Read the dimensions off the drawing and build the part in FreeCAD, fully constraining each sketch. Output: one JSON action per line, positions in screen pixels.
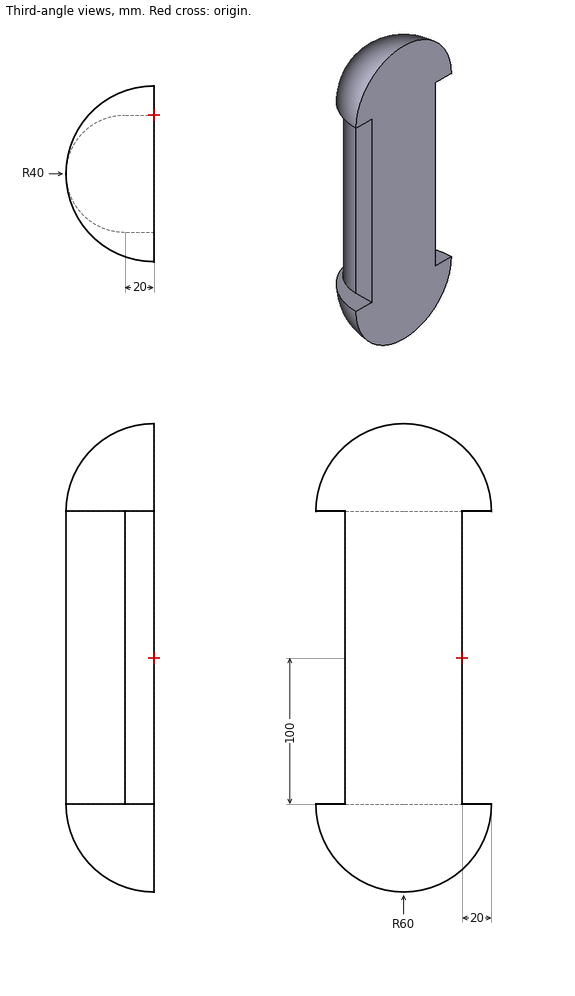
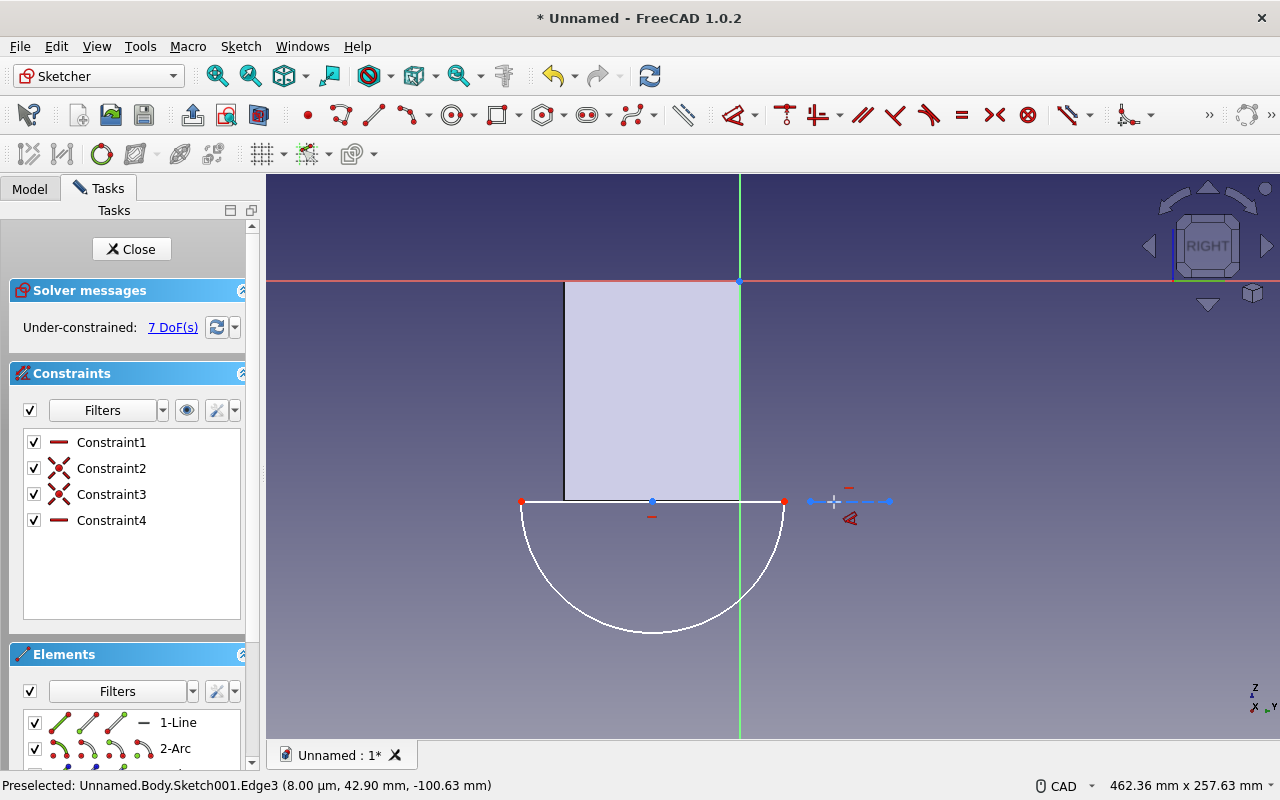
{"action": "left_click", "coordinate": [575, 608]}
{"action": "left_click", "coordinate": [556, 634]}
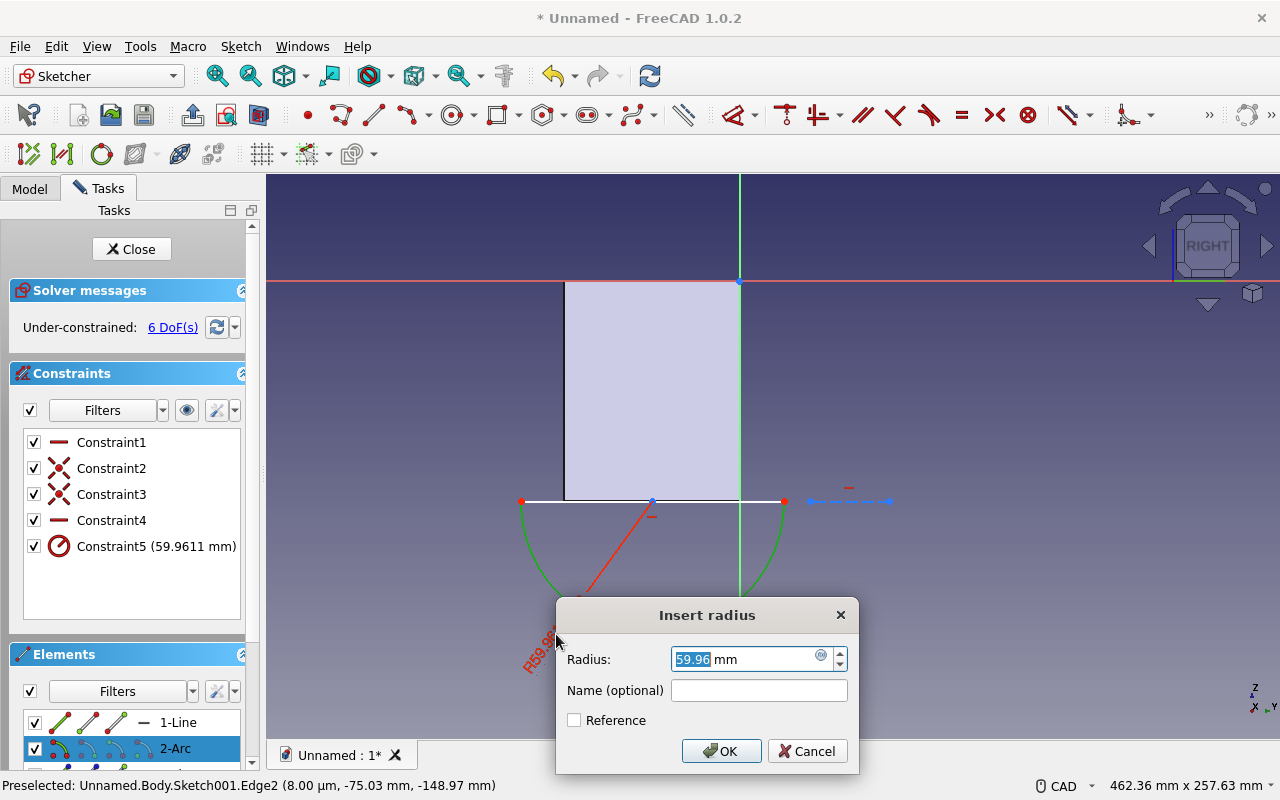
{"action": "type", "text": "60"}
{"action": "key", "text": "Return"}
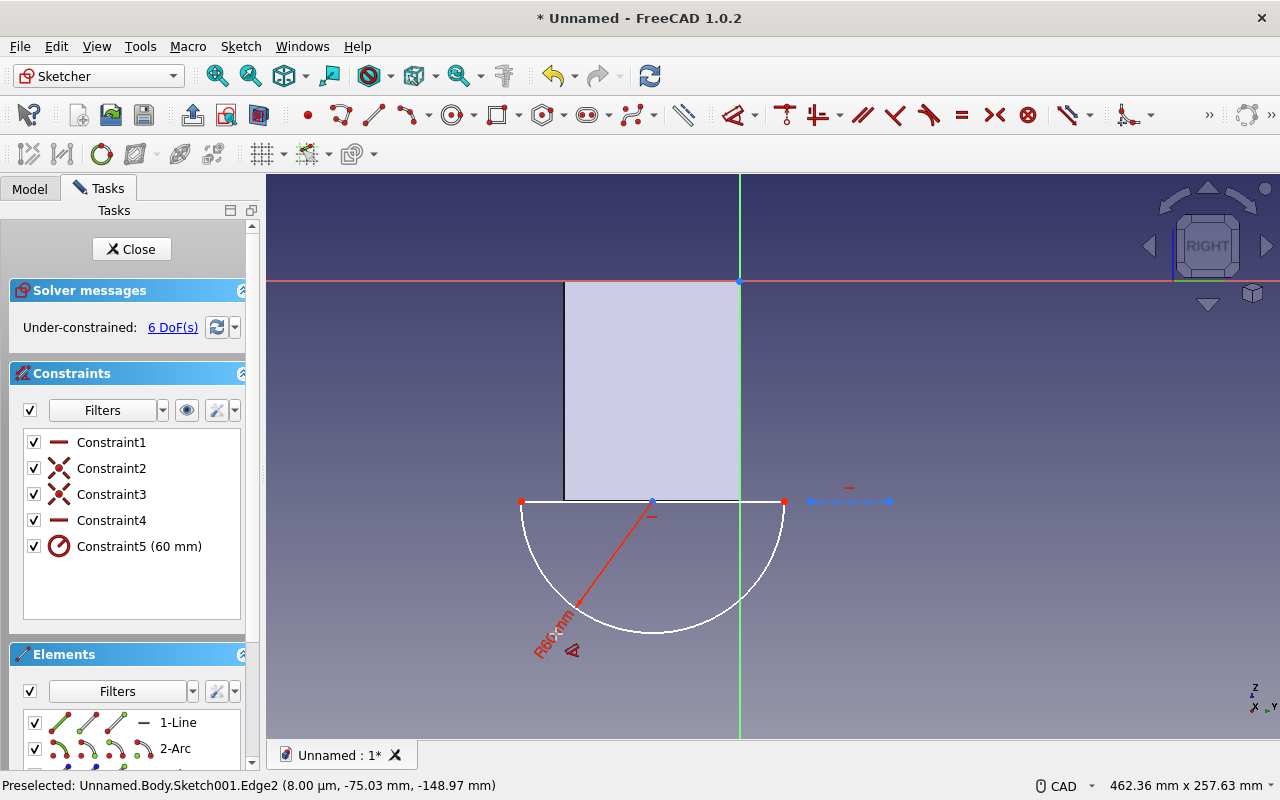
{"action": "left_click", "coordinate": [784, 502]}
{"action": "left_click", "coordinate": [762, 247]}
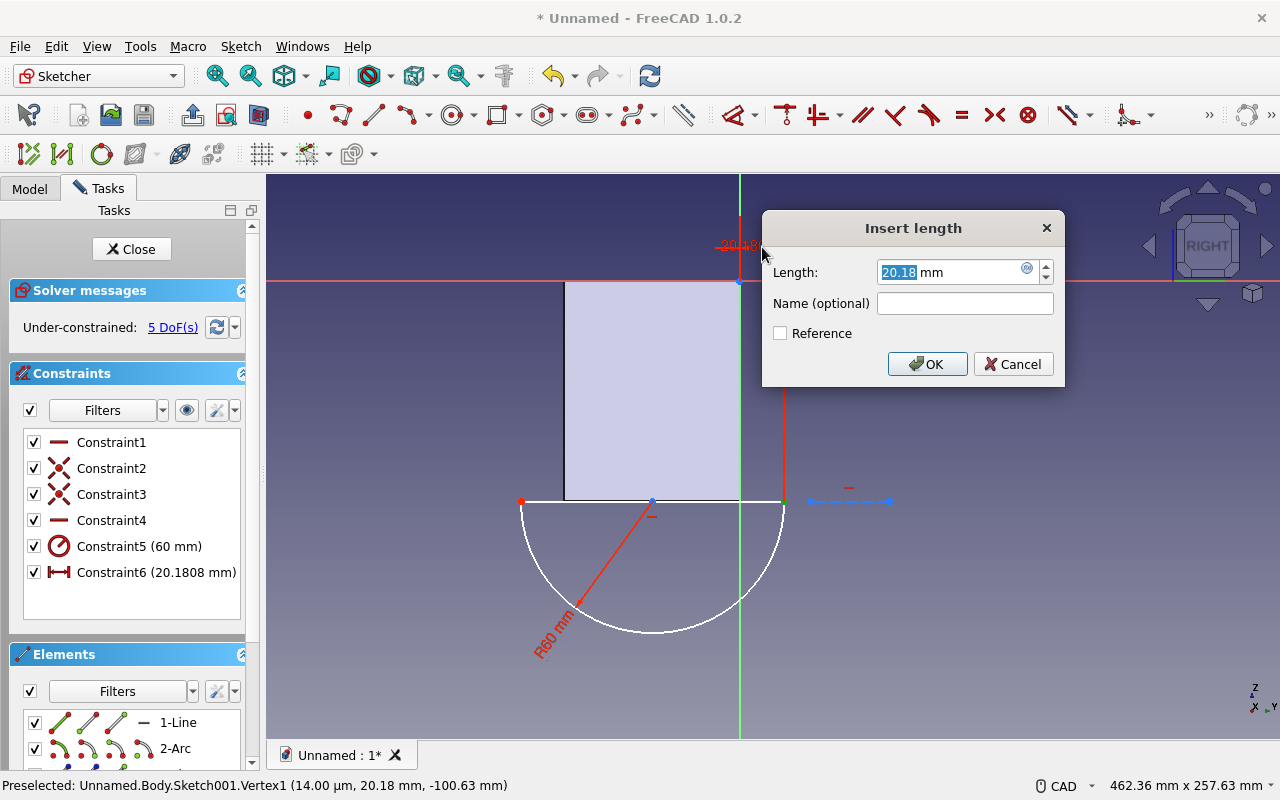
{"action": "type", "text": "20"}
{"action": "key", "text": "Return"}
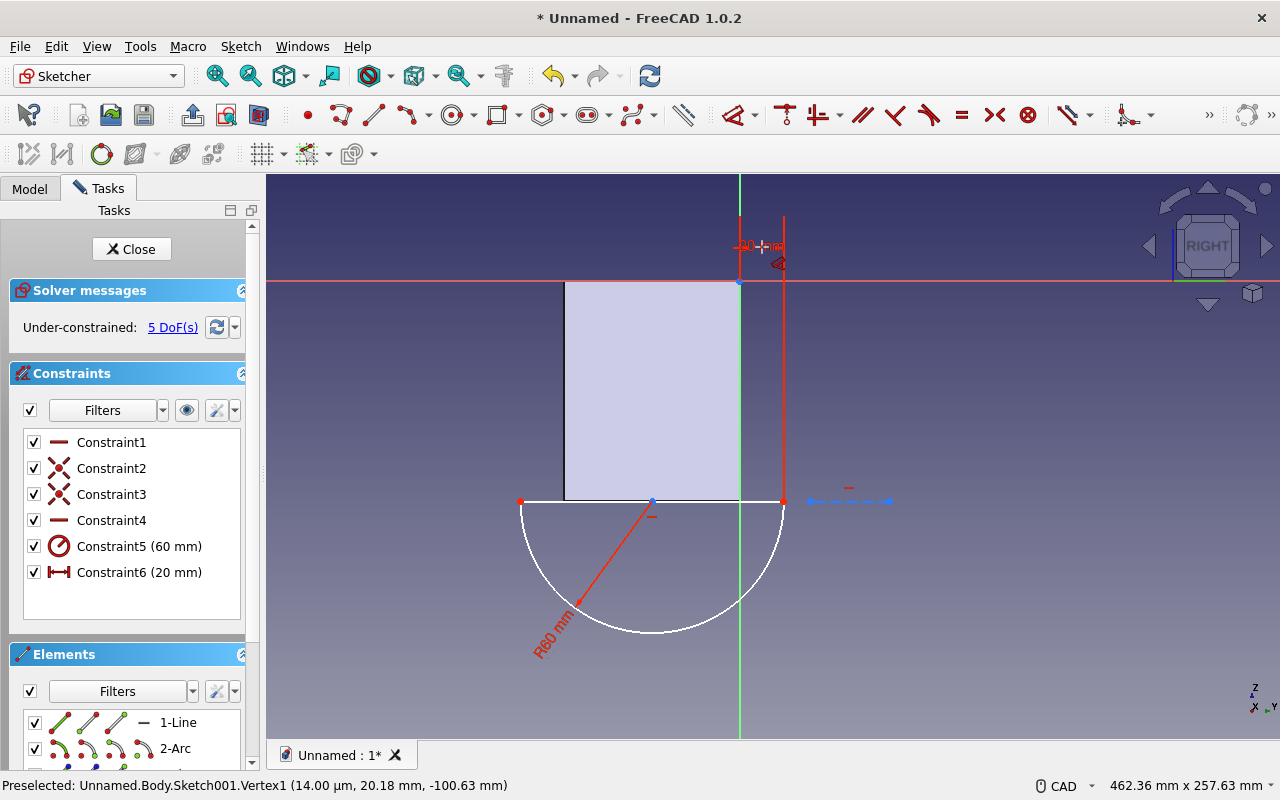
{"action": "left_click", "coordinate": [784, 502]}
{"action": "left_click", "coordinate": [818, 392]}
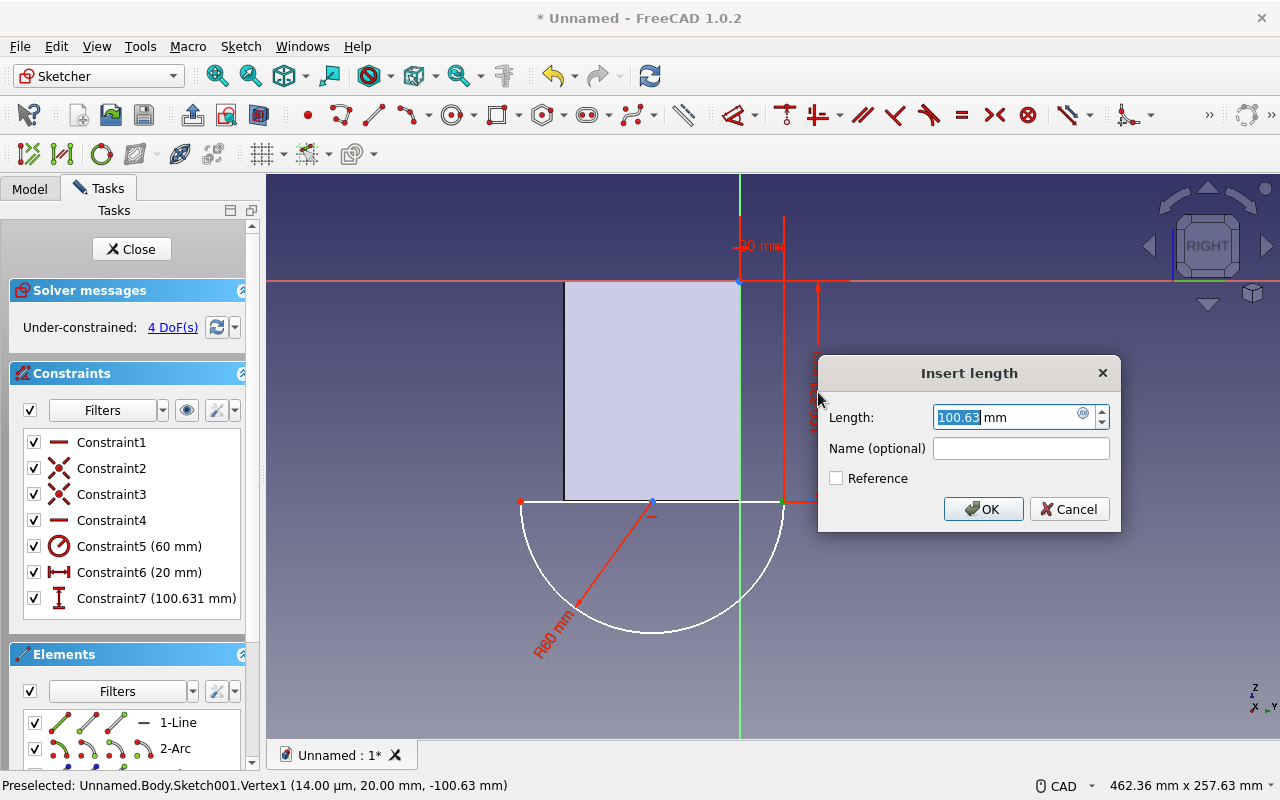
{"action": "type", "text": "100"}
{"action": "key", "text": "Return"}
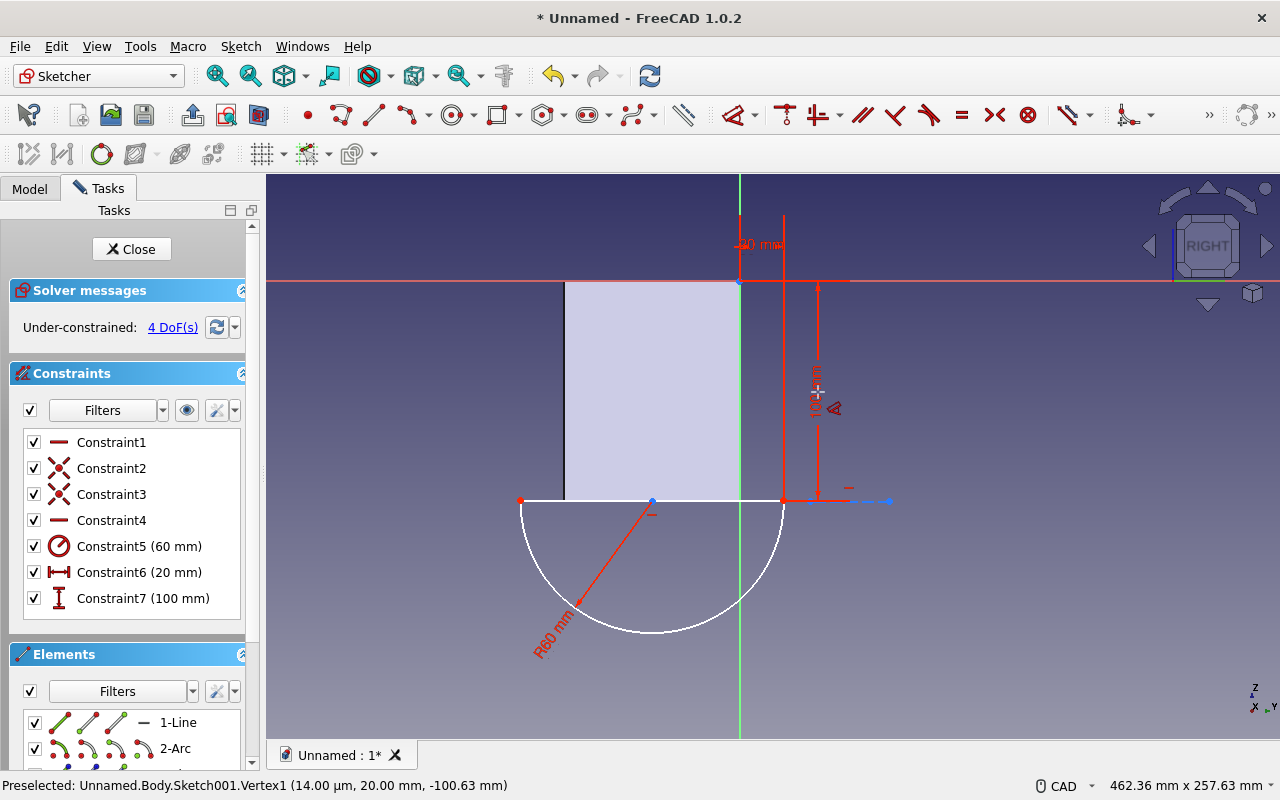
{"action": "left_click", "coordinate": [810, 502]}
{"action": "left_click", "coordinate": [844, 341]}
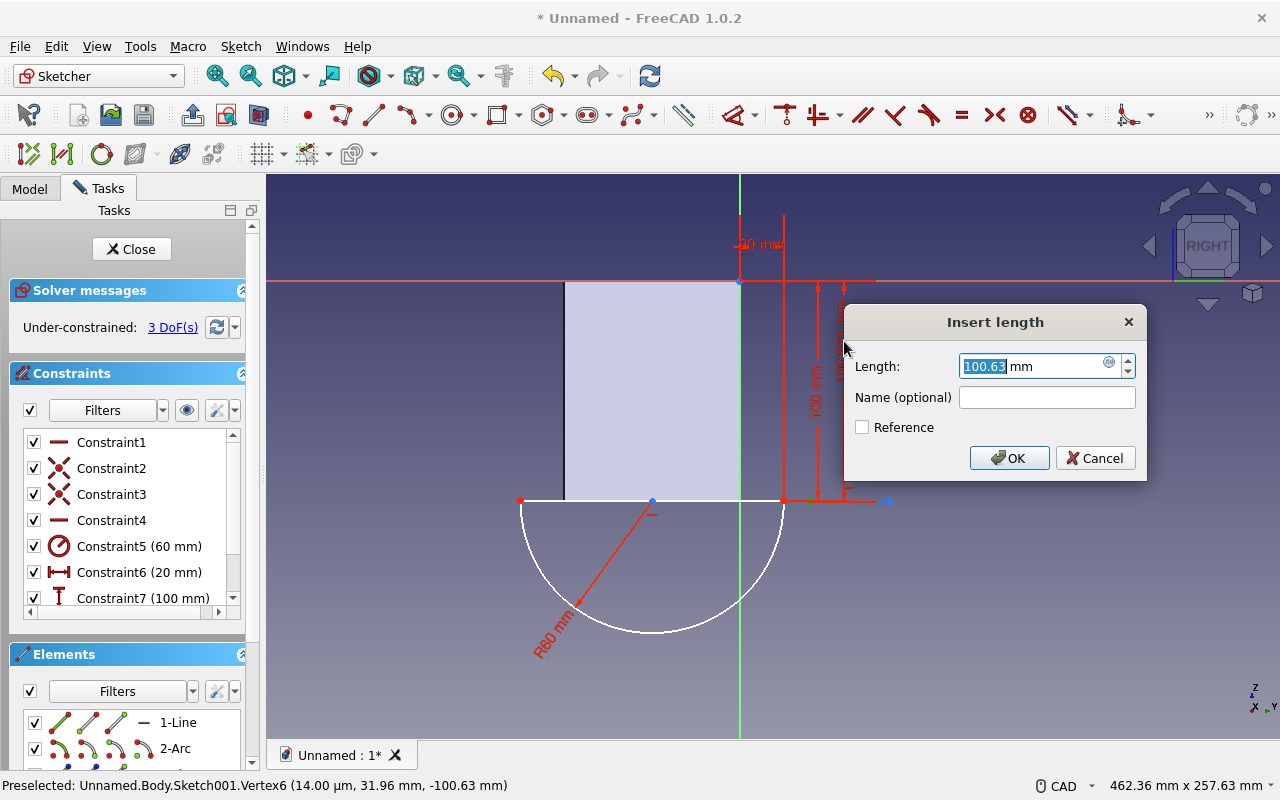
{"action": "type", "text": "100"}
{"action": "key", "text": "Return"}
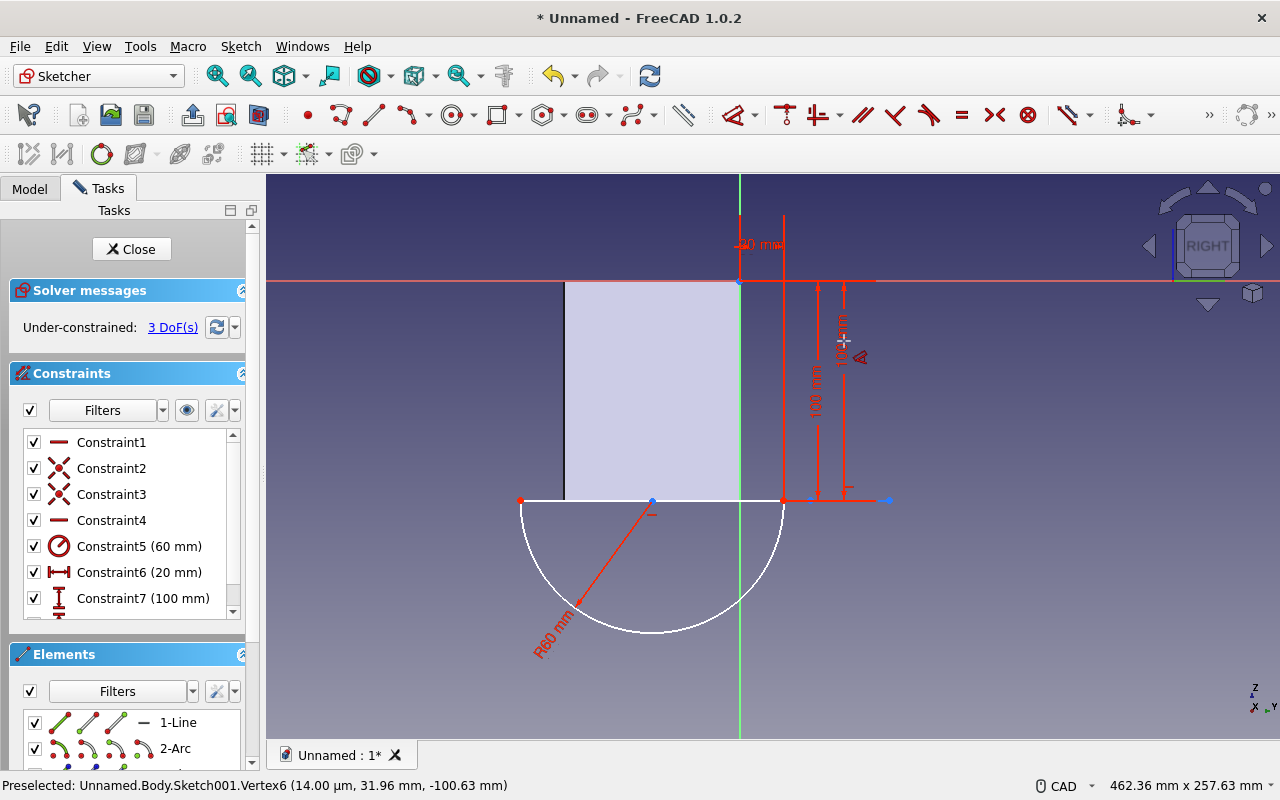
{"action": "left_click", "coordinate": [652, 501]}
{"action": "left_click", "coordinate": [618, 391]}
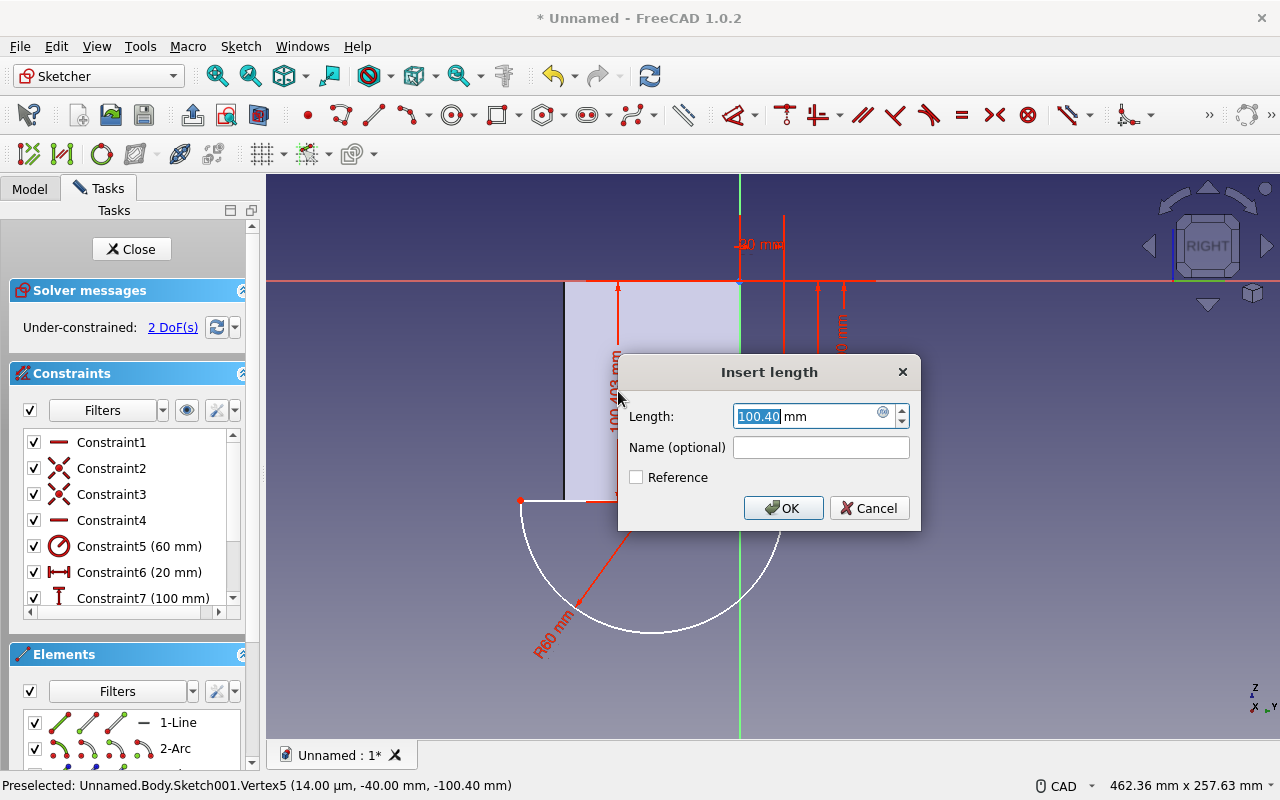
{"action": "type", "text": "100"}
{"action": "key", "text": "Return"}
{"action": "key", "text": "Escape"}